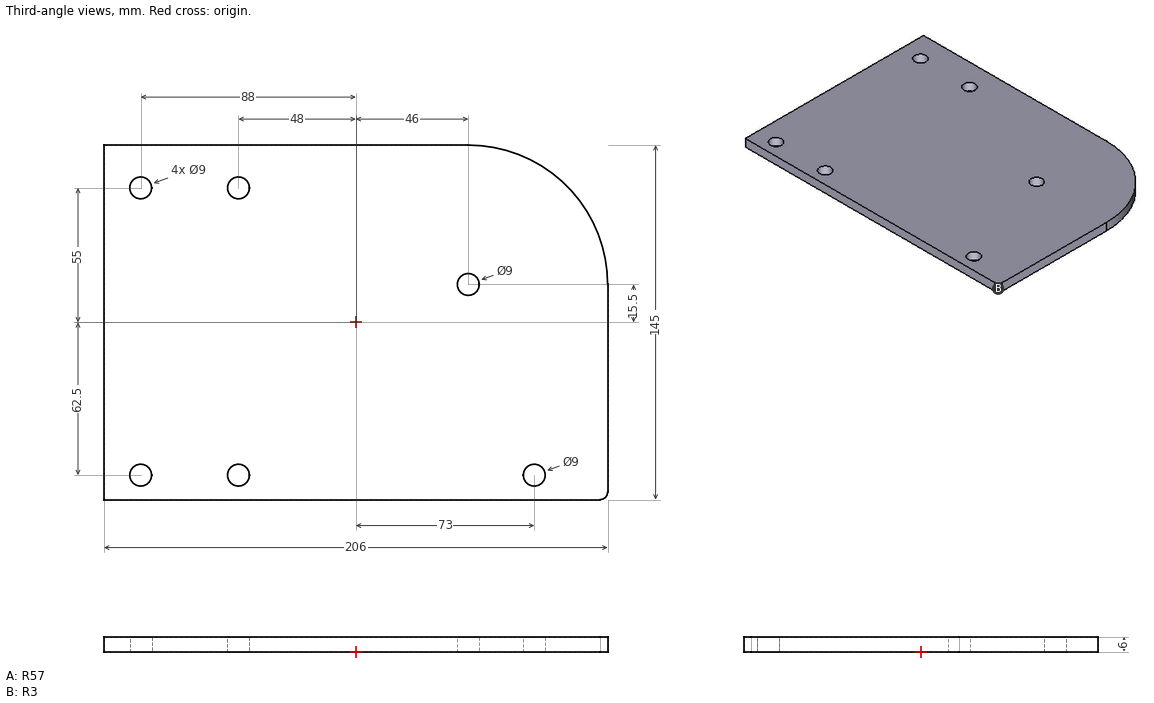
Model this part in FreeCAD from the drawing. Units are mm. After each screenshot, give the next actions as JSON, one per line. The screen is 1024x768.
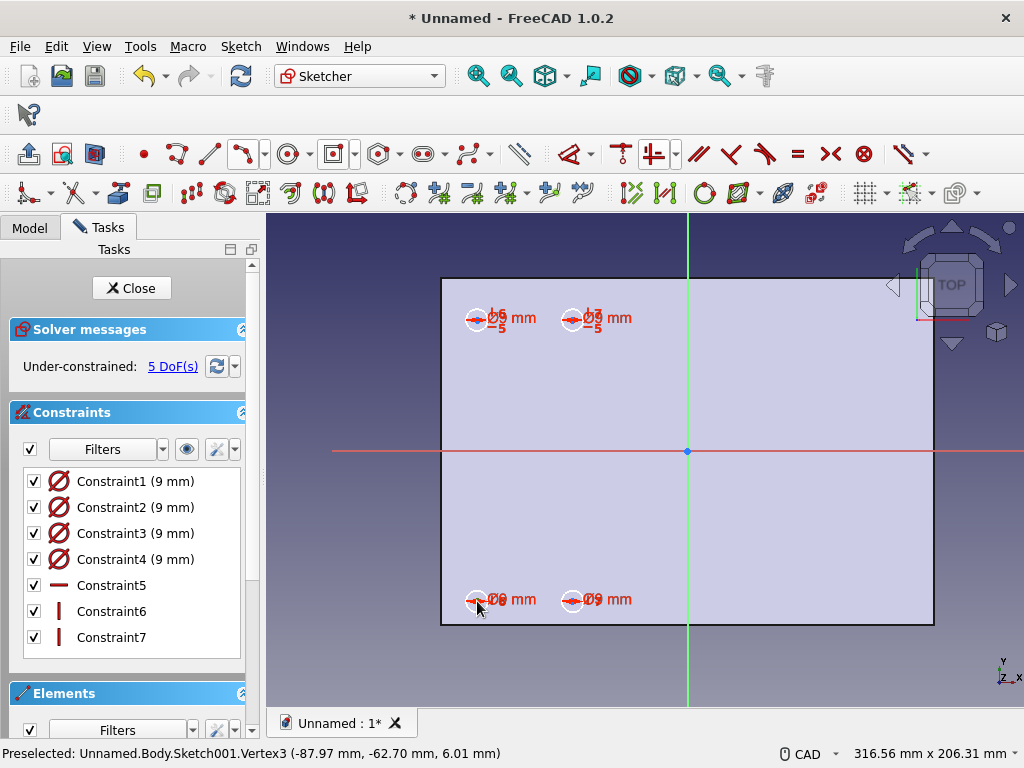
{"action": "left_click", "coordinate": [573, 601]}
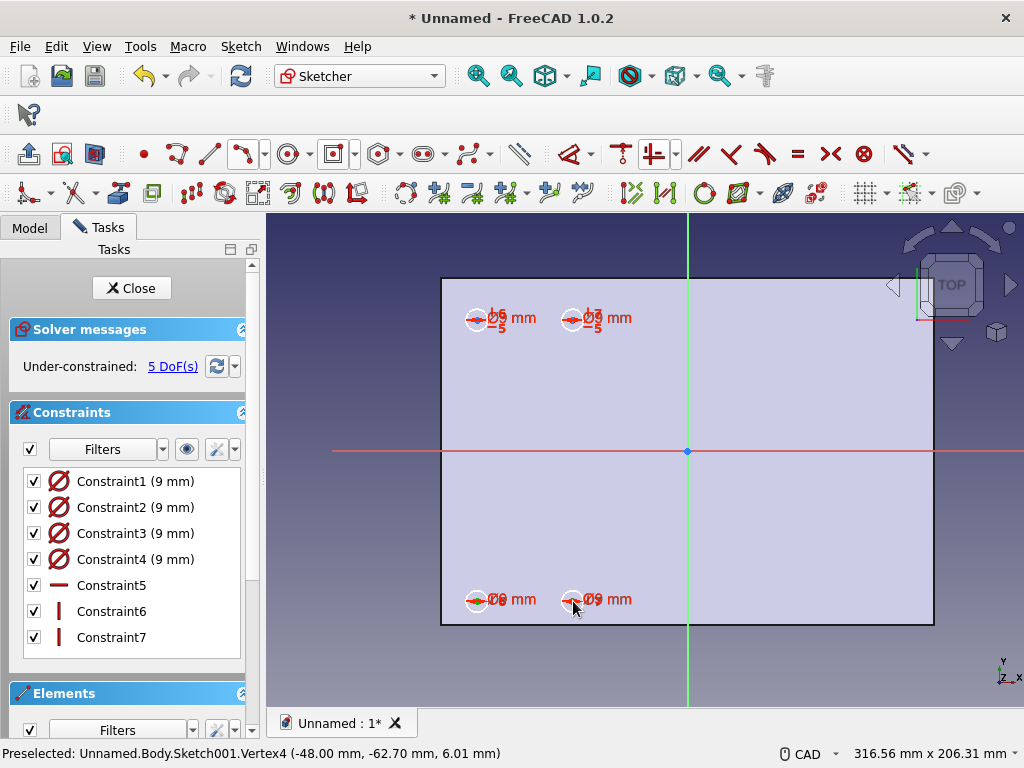
{"action": "key", "text": "h"}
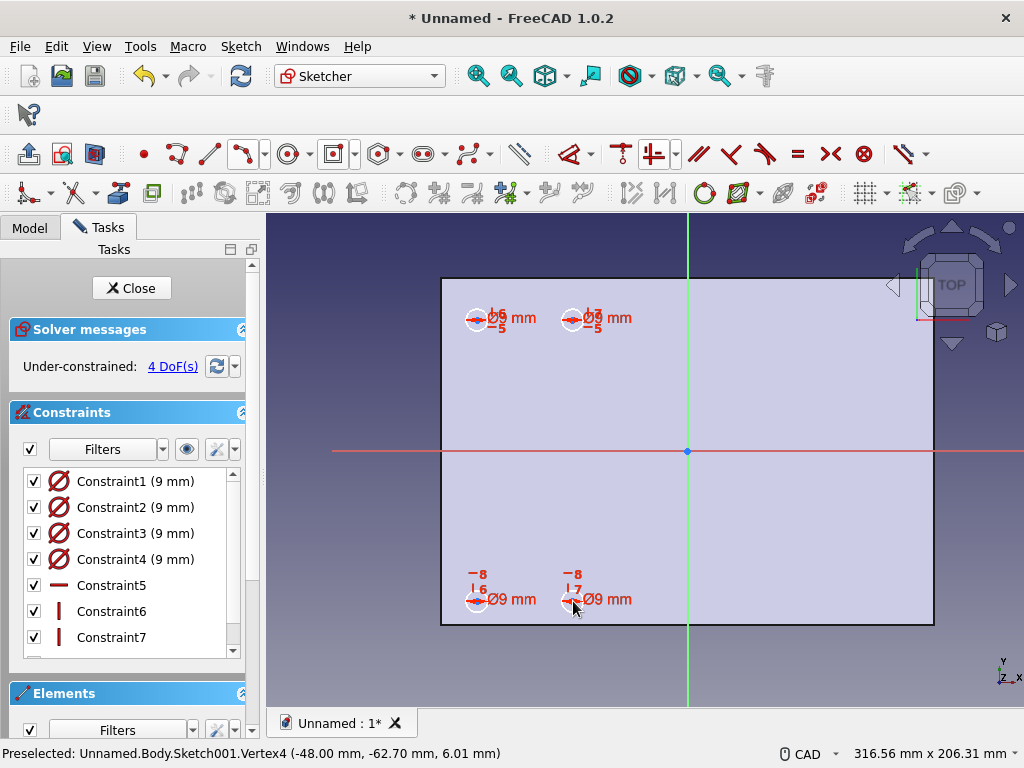
{"action": "left_click", "coordinate": [568, 154]}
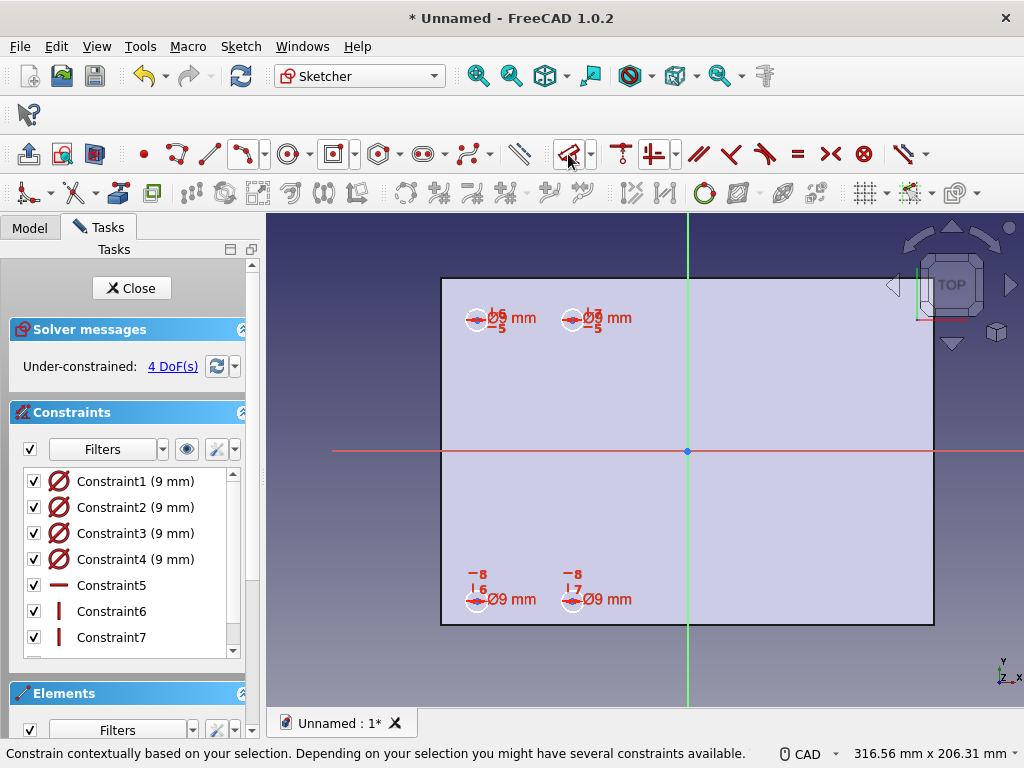
{"action": "left_click", "coordinate": [477, 320]}
{"action": "left_click", "coordinate": [582, 286]}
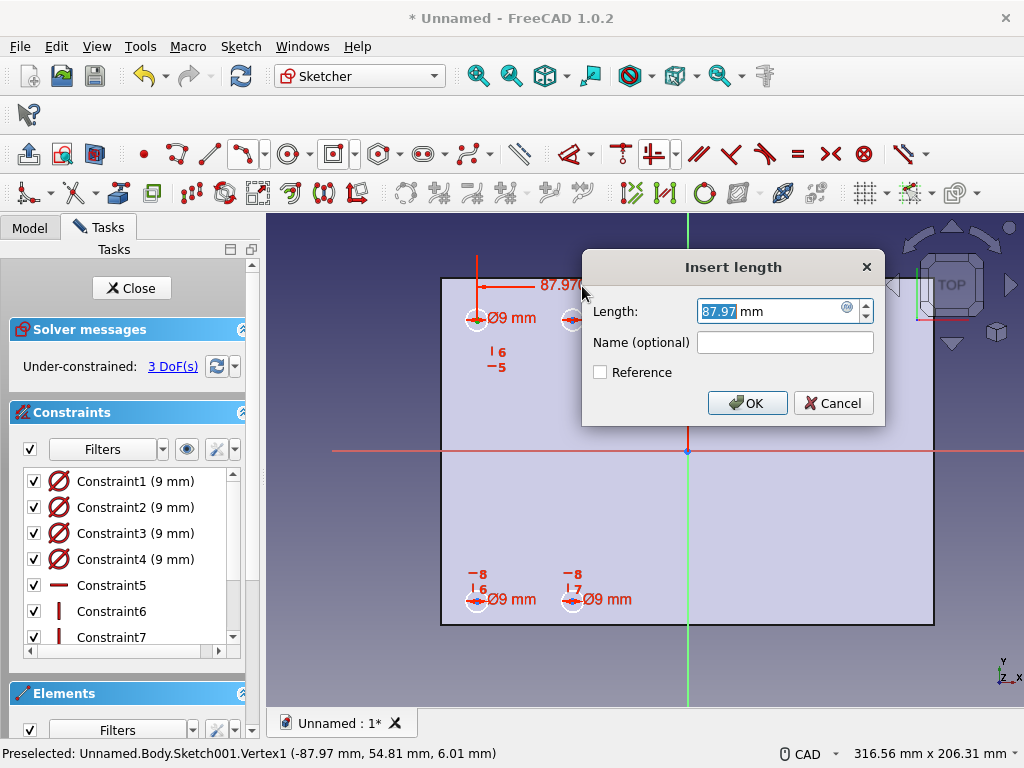
{"action": "type", "text": "88"}
{"action": "key", "text": "Return"}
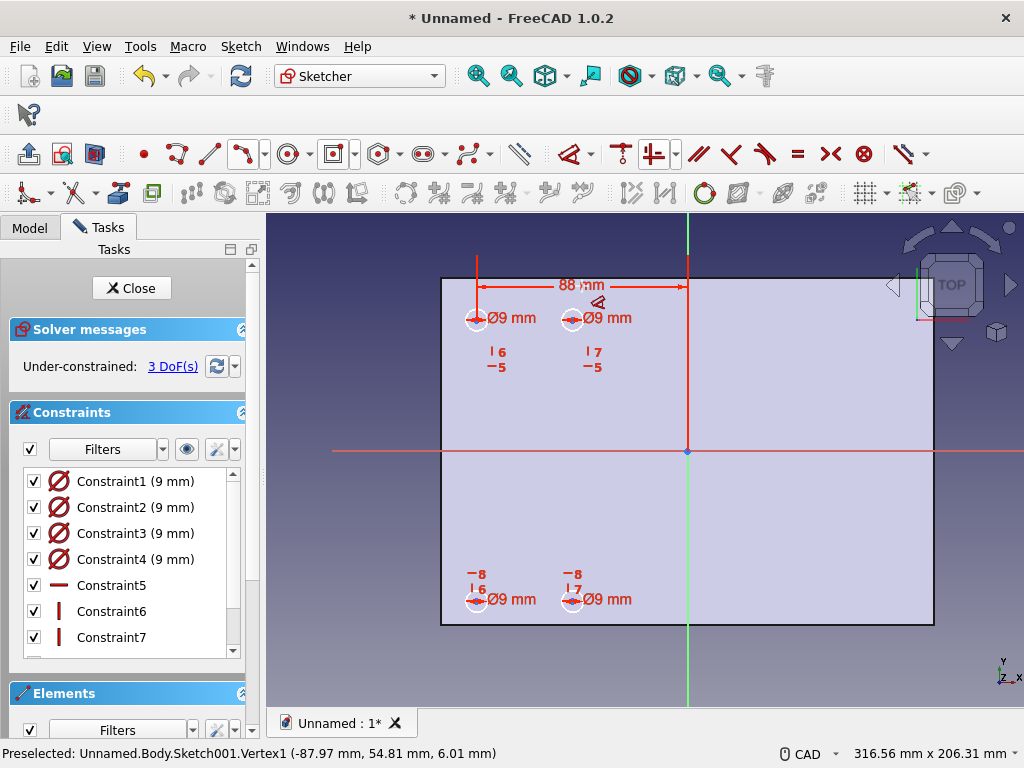
{"action": "left_click", "coordinate": [477, 320]}
{"action": "left_click", "coordinate": [722, 386]}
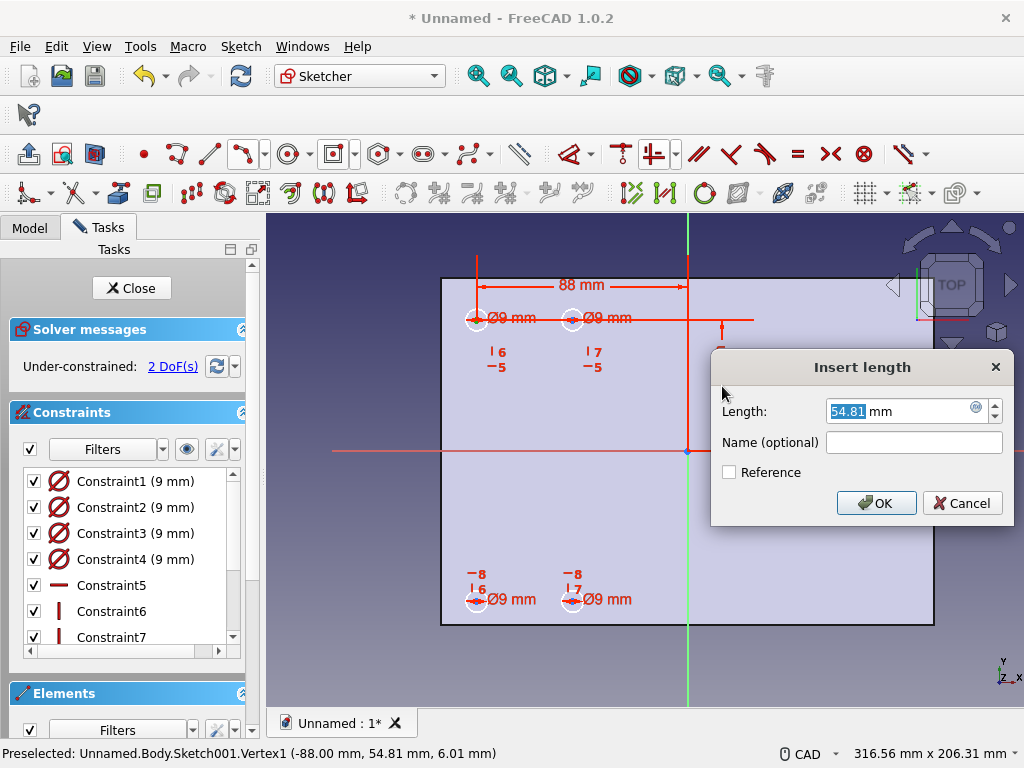
{"action": "type", "text": "55"}
{"action": "key", "text": "Return"}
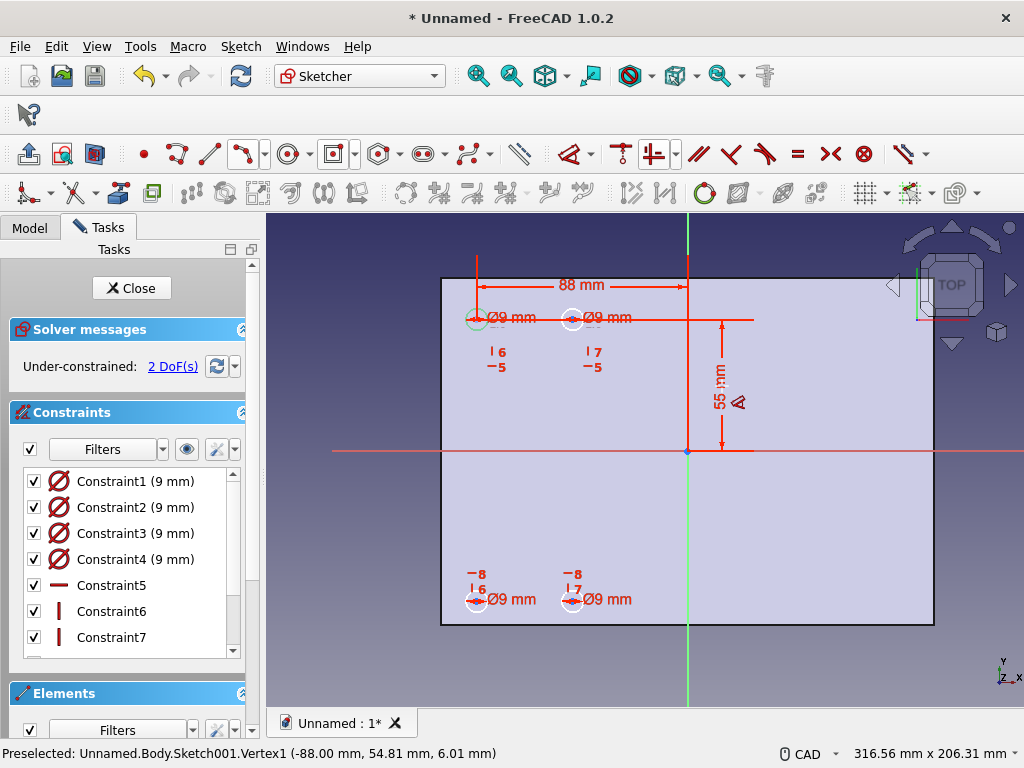
{"action": "left_click", "coordinate": [573, 320]}
{"action": "left_click", "coordinate": [657, 286]}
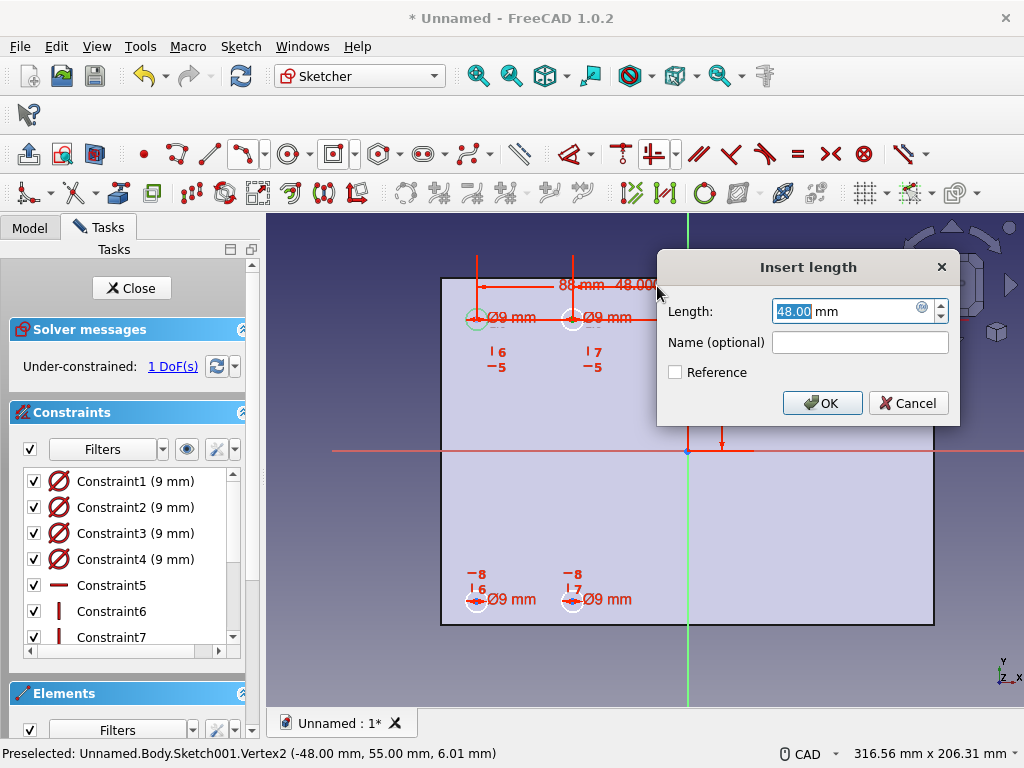
{"action": "type", "text": "48"}
{"action": "key", "text": "Return"}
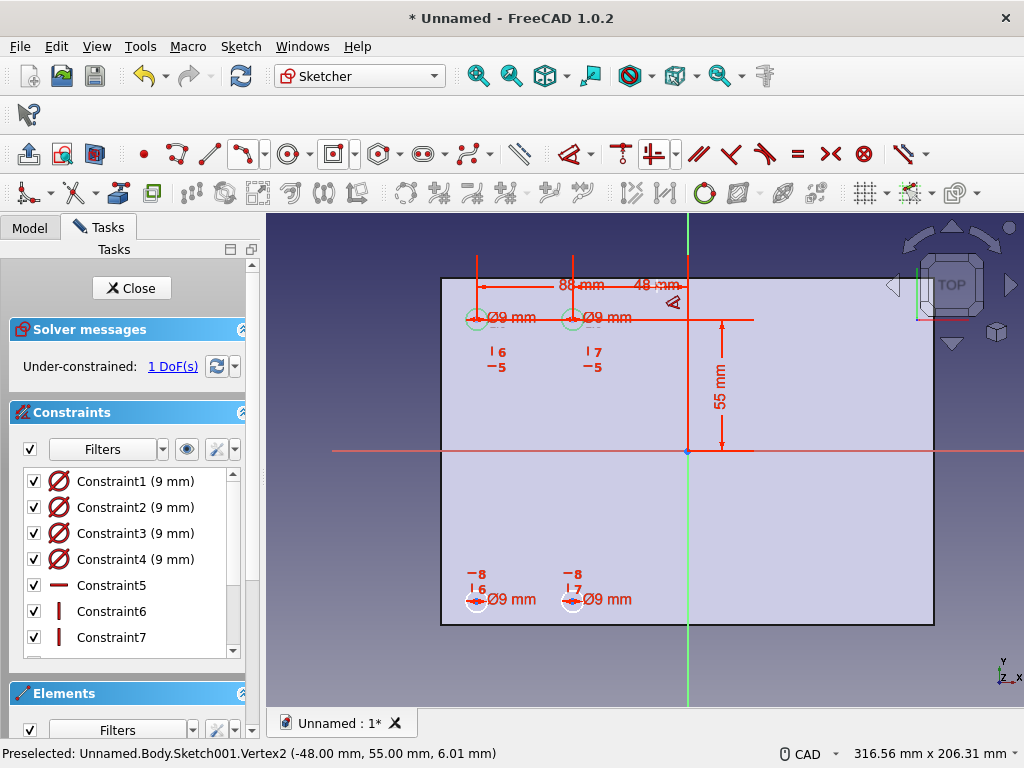
{"action": "left_click", "coordinate": [477, 601]}
{"action": "left_click", "coordinate": [722, 526]}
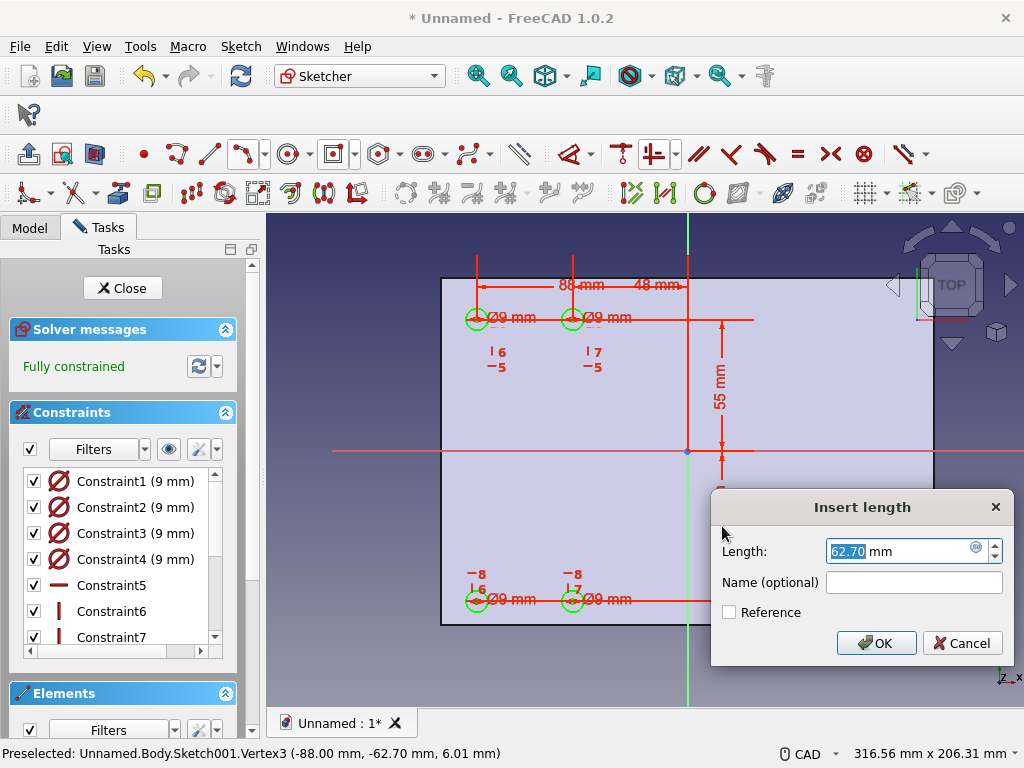
{"action": "type", "text": "62.5"}
{"action": "key", "text": "Return"}
{"action": "key", "text": "Escape"}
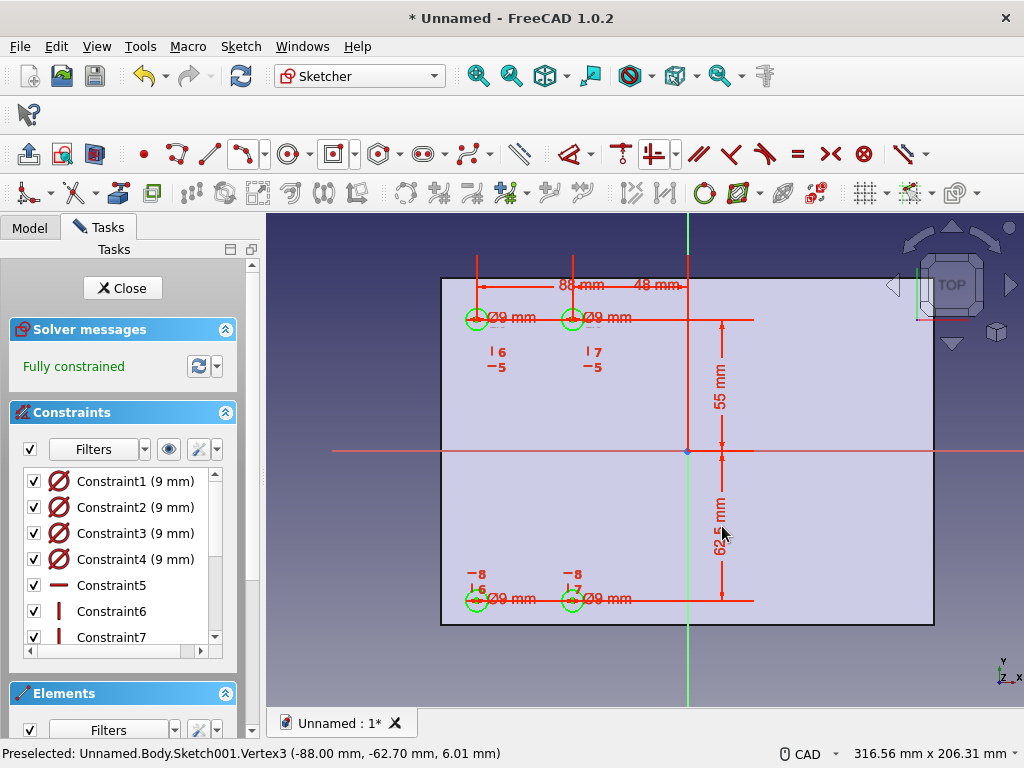
{"action": "left_click", "coordinate": [123, 288]}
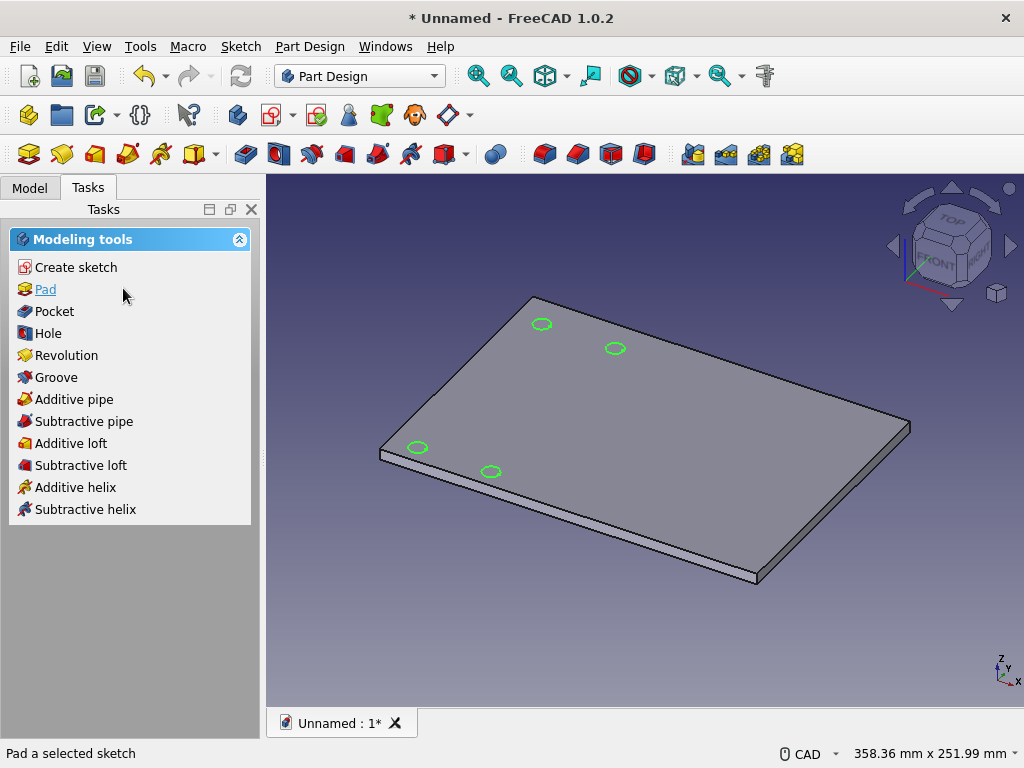
{"action": "left_click", "coordinate": [246, 154]}